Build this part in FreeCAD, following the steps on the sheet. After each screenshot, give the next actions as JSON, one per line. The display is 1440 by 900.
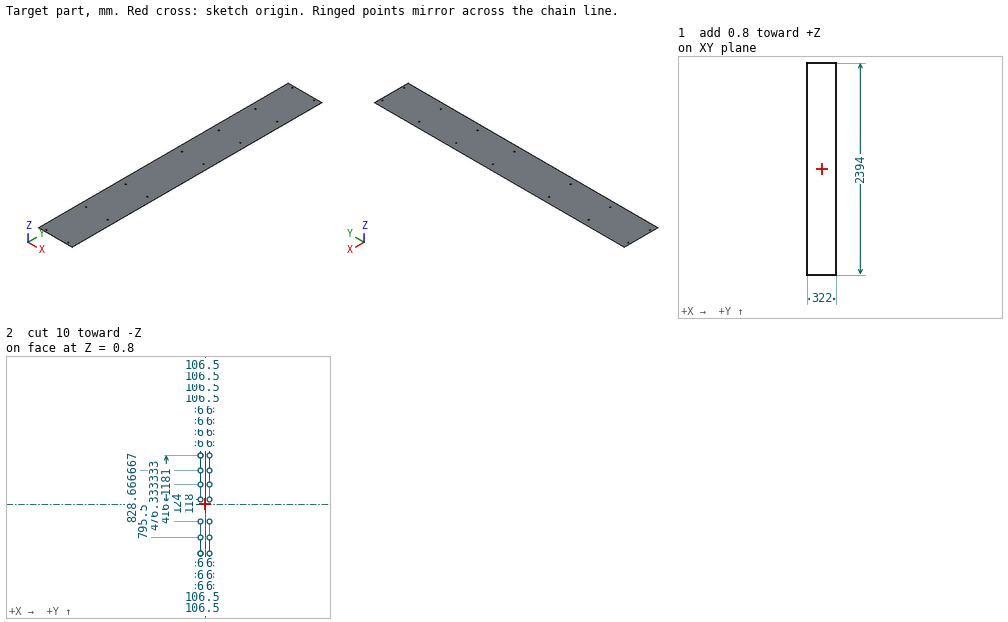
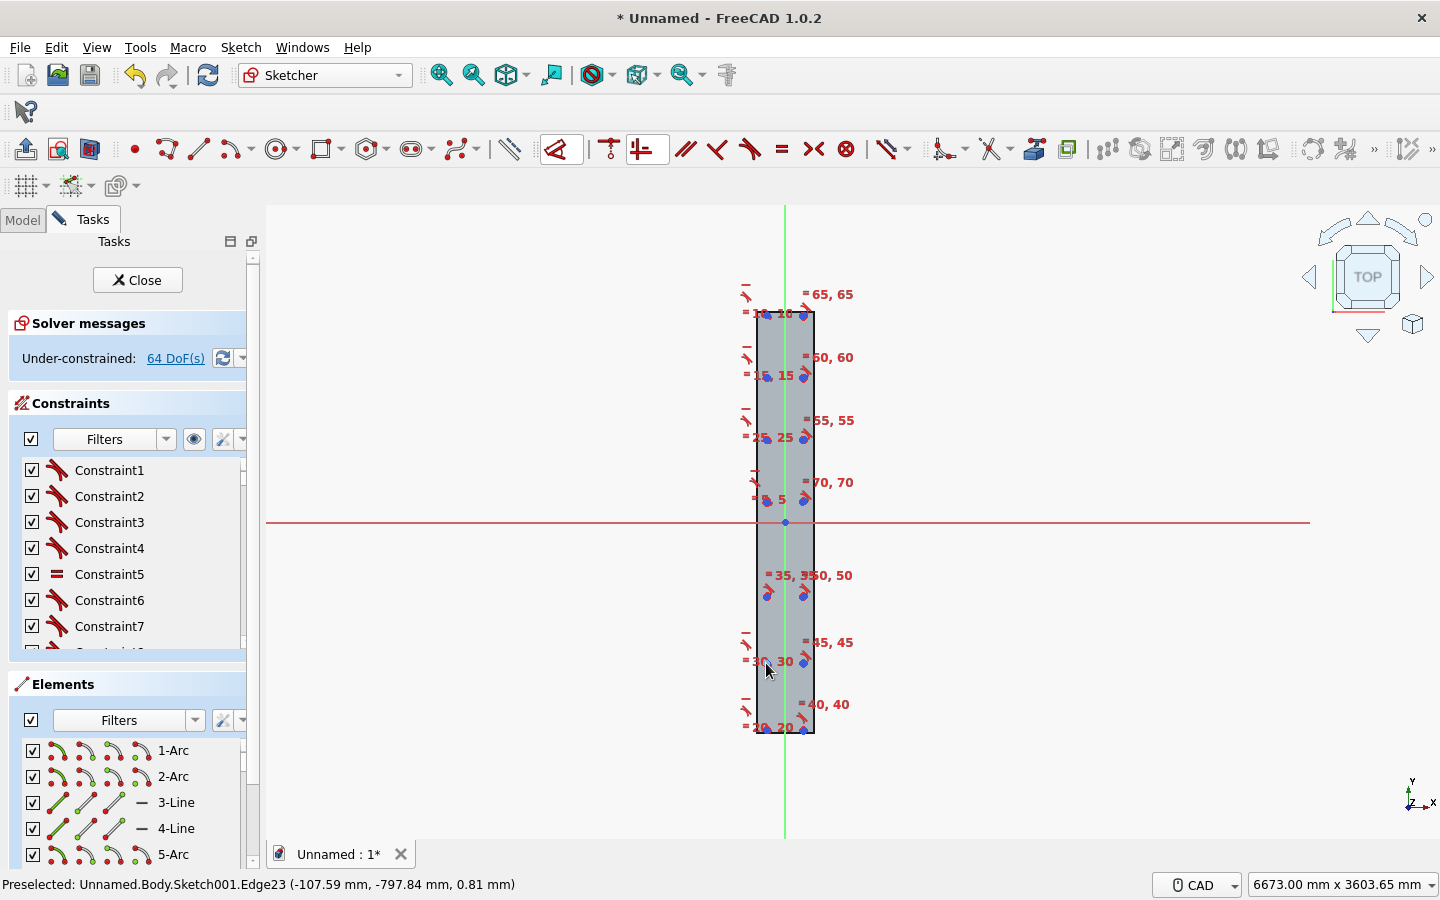
{"action": "scroll", "coordinate": [767, 596], "scroll_direction": "up", "scroll_amount": 14}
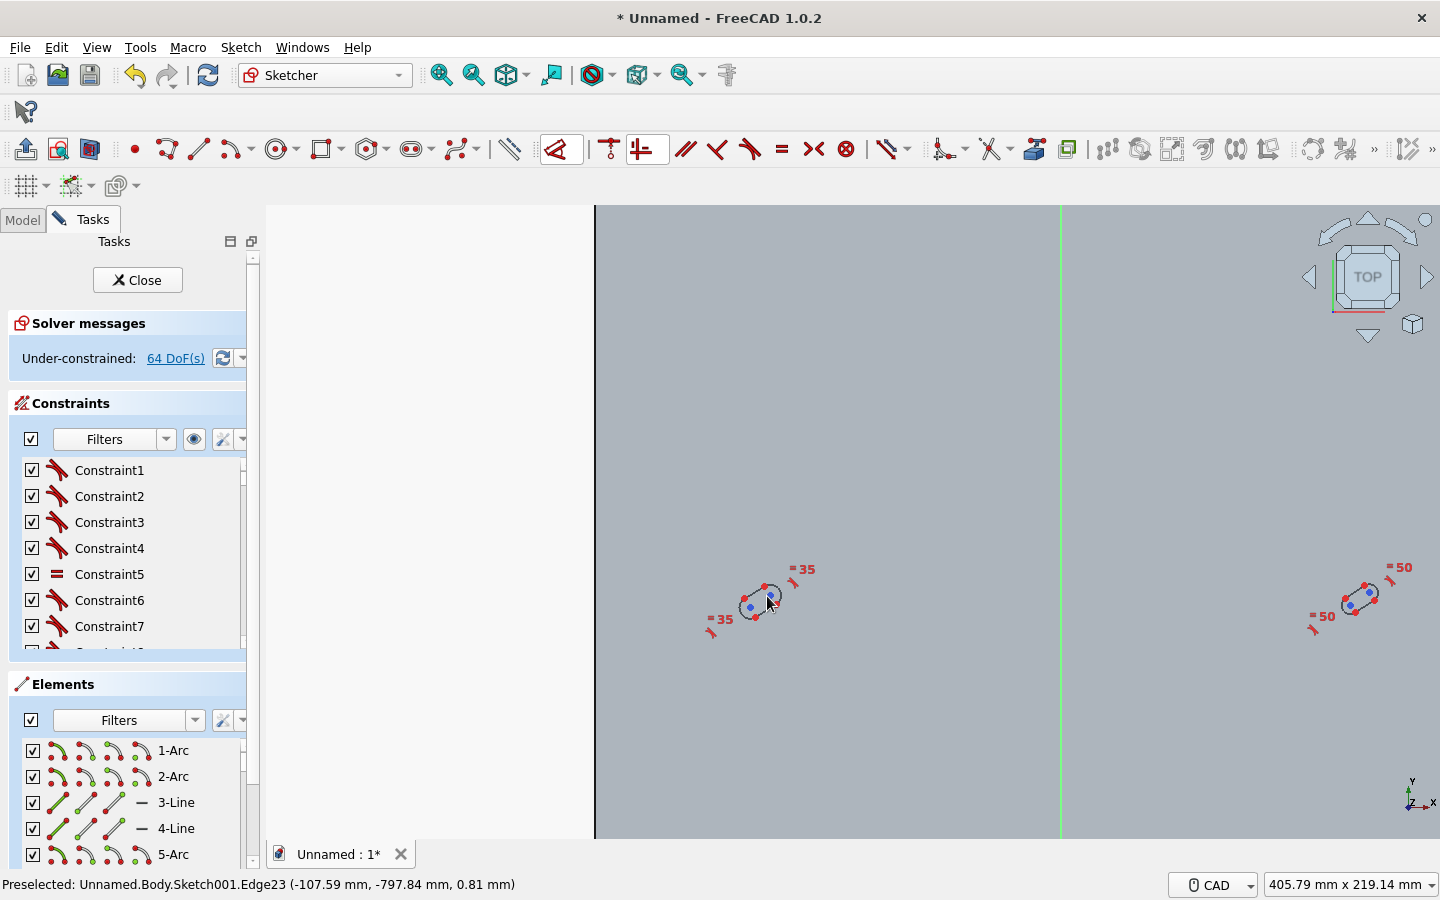
{"action": "left_click", "coordinate": [753, 594]}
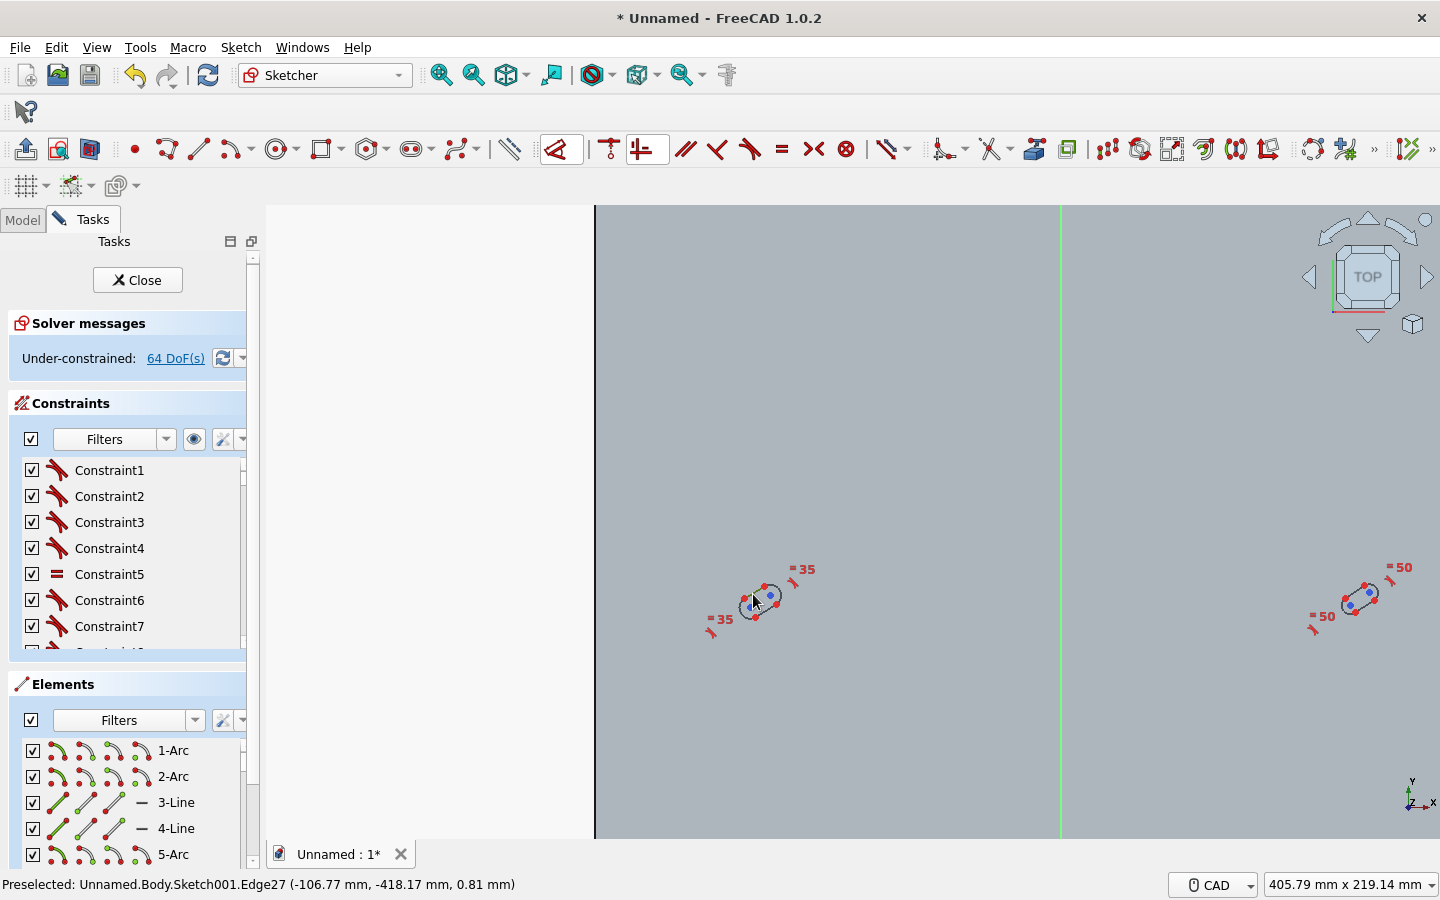
{"action": "key", "text": "h"}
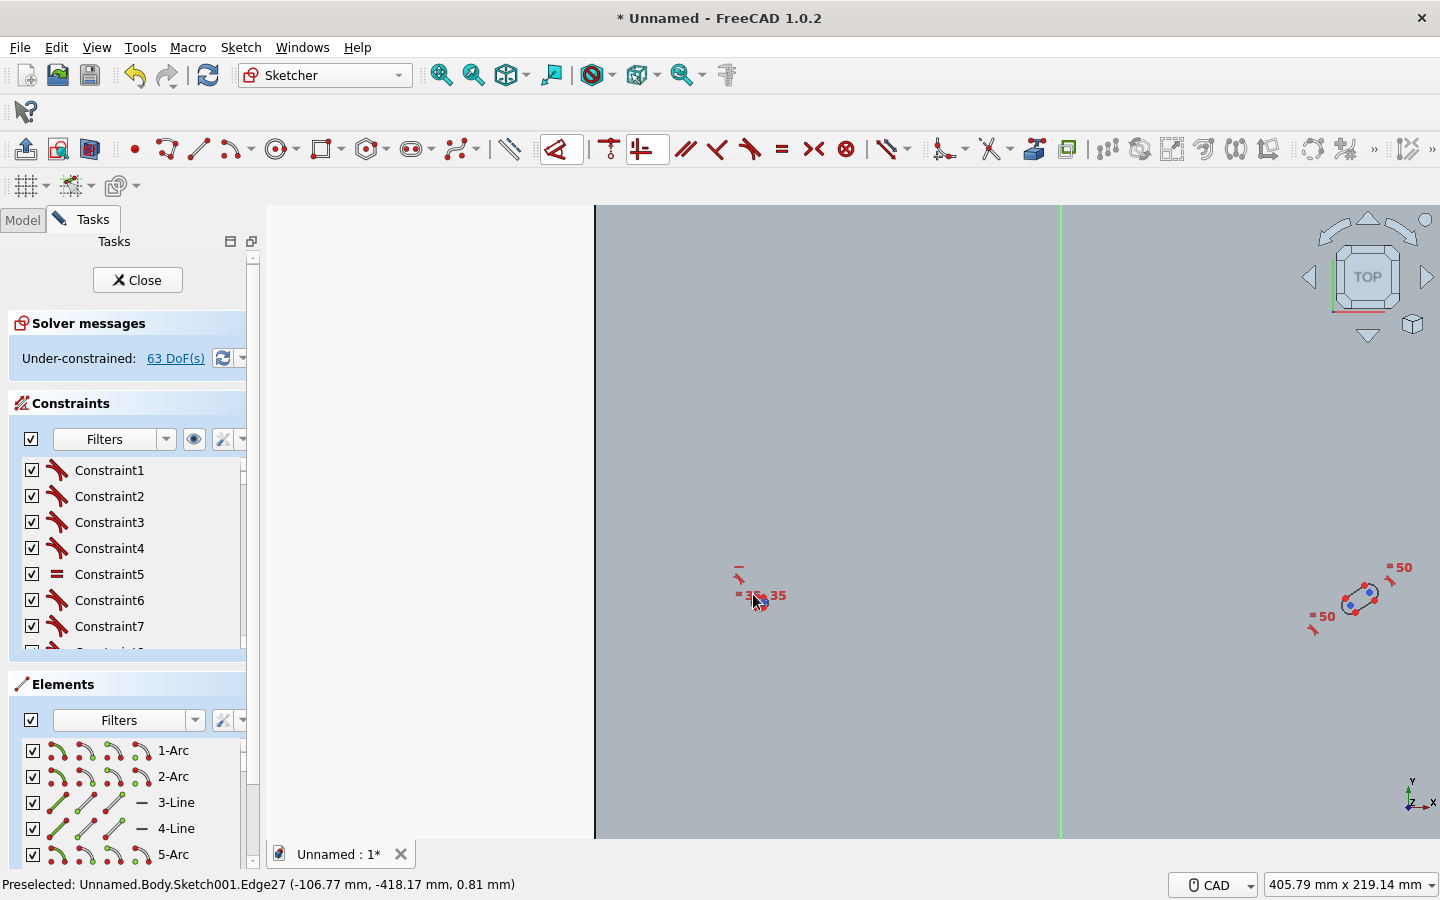
{"action": "scroll", "coordinate": [767, 596], "scroll_direction": "down", "scroll_amount": 14}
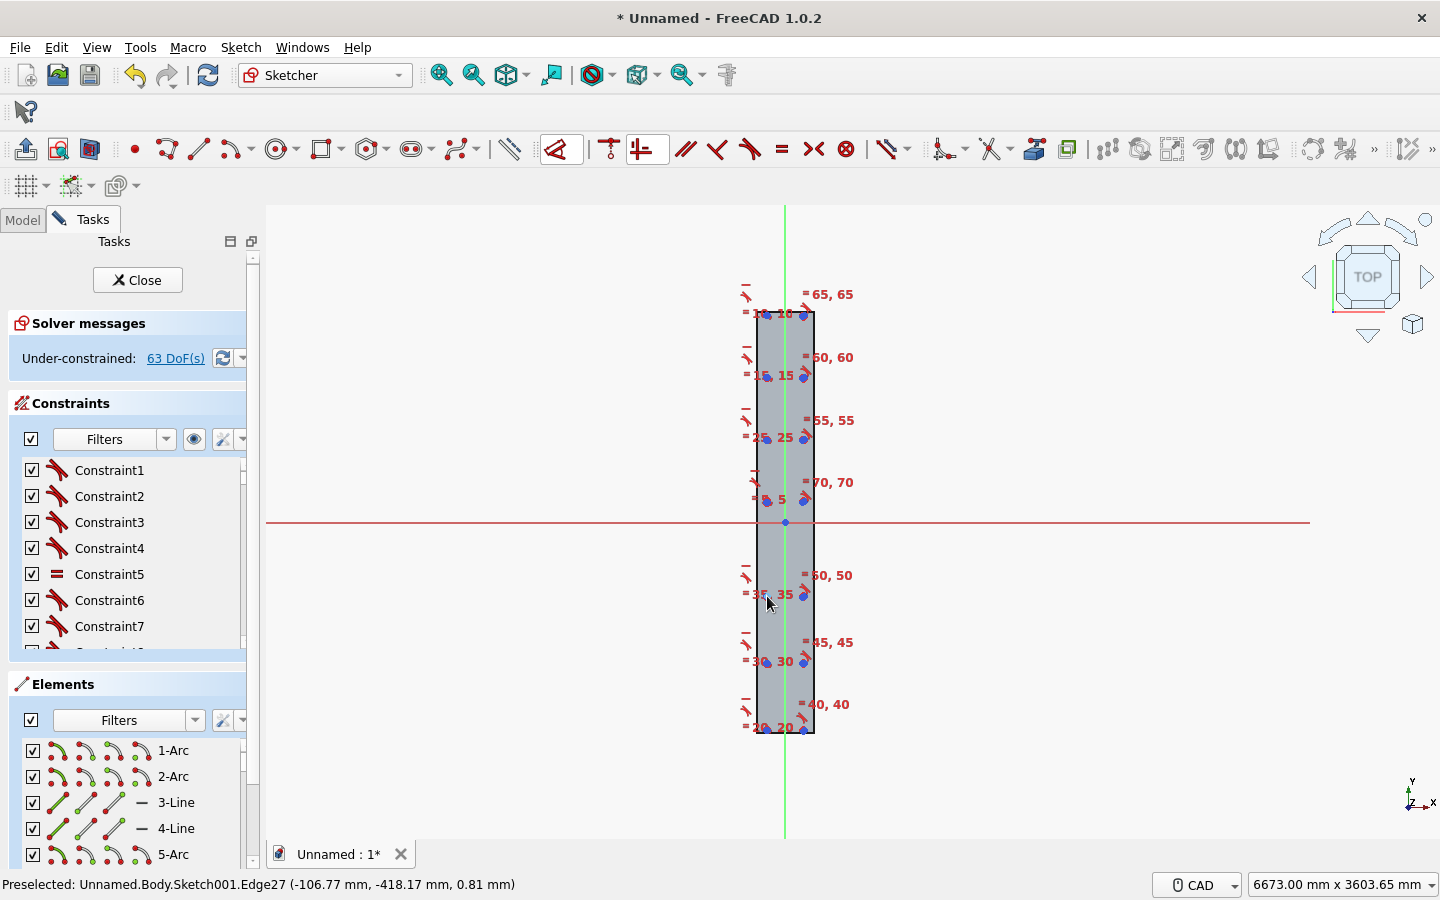
{"action": "scroll", "coordinate": [803, 730], "scroll_direction": "up", "scroll_amount": 14}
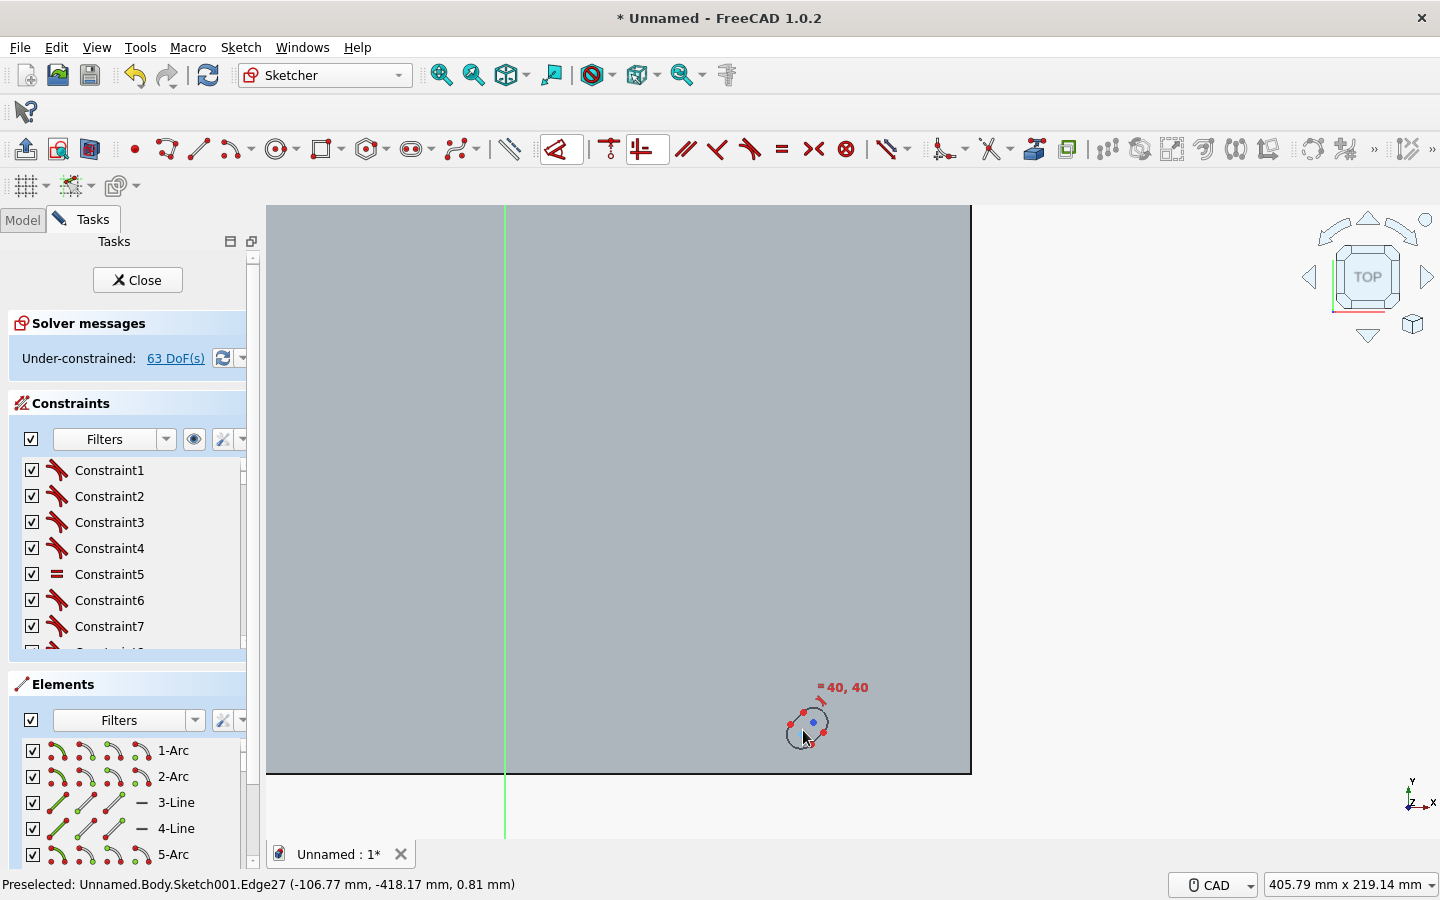
{"action": "left_click", "coordinate": [797, 718]}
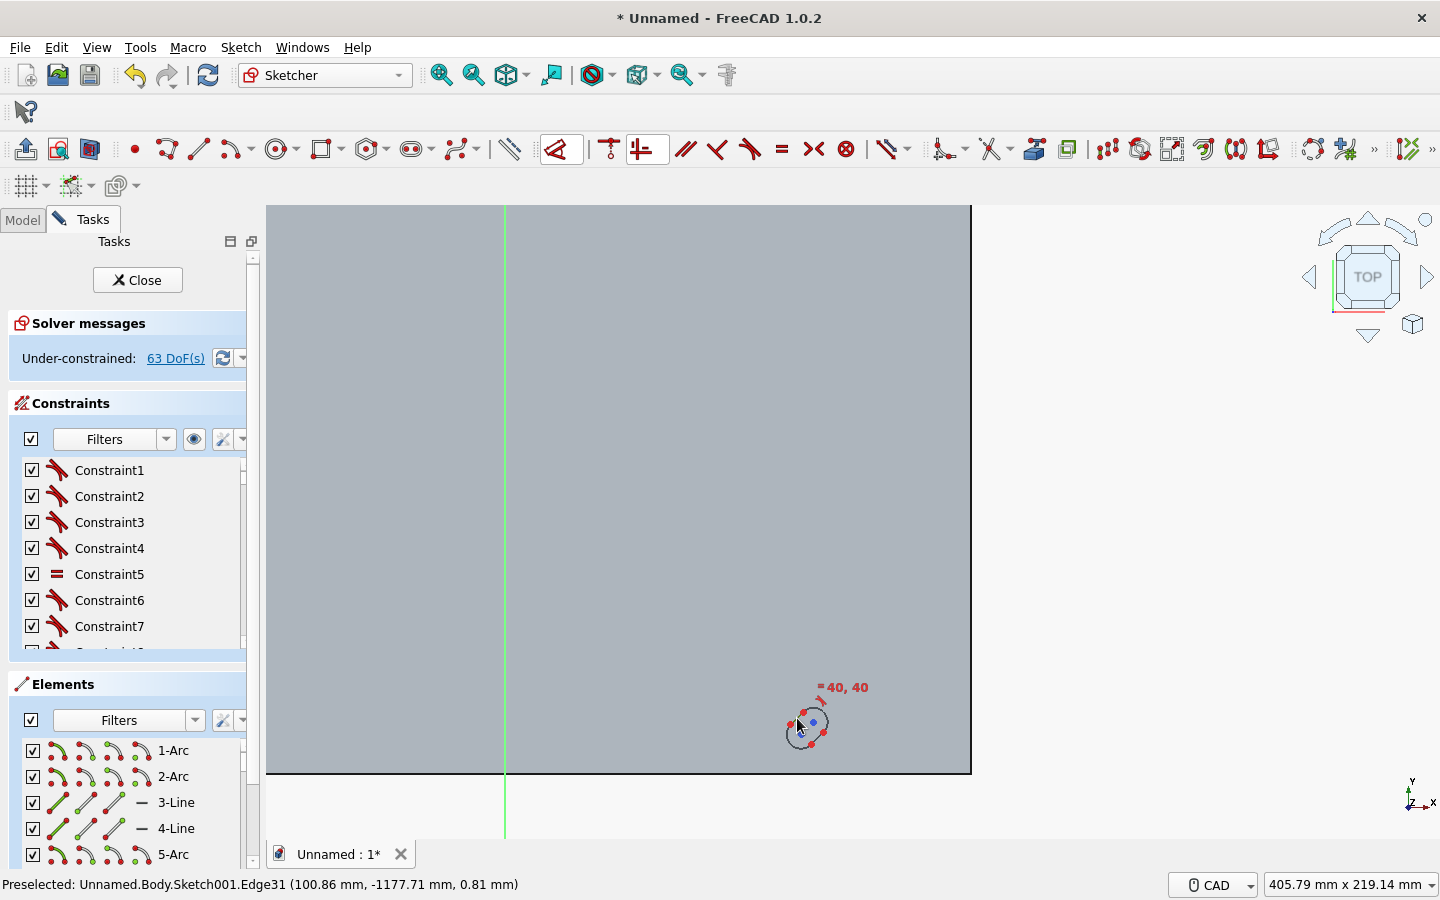
{"action": "key", "text": "h"}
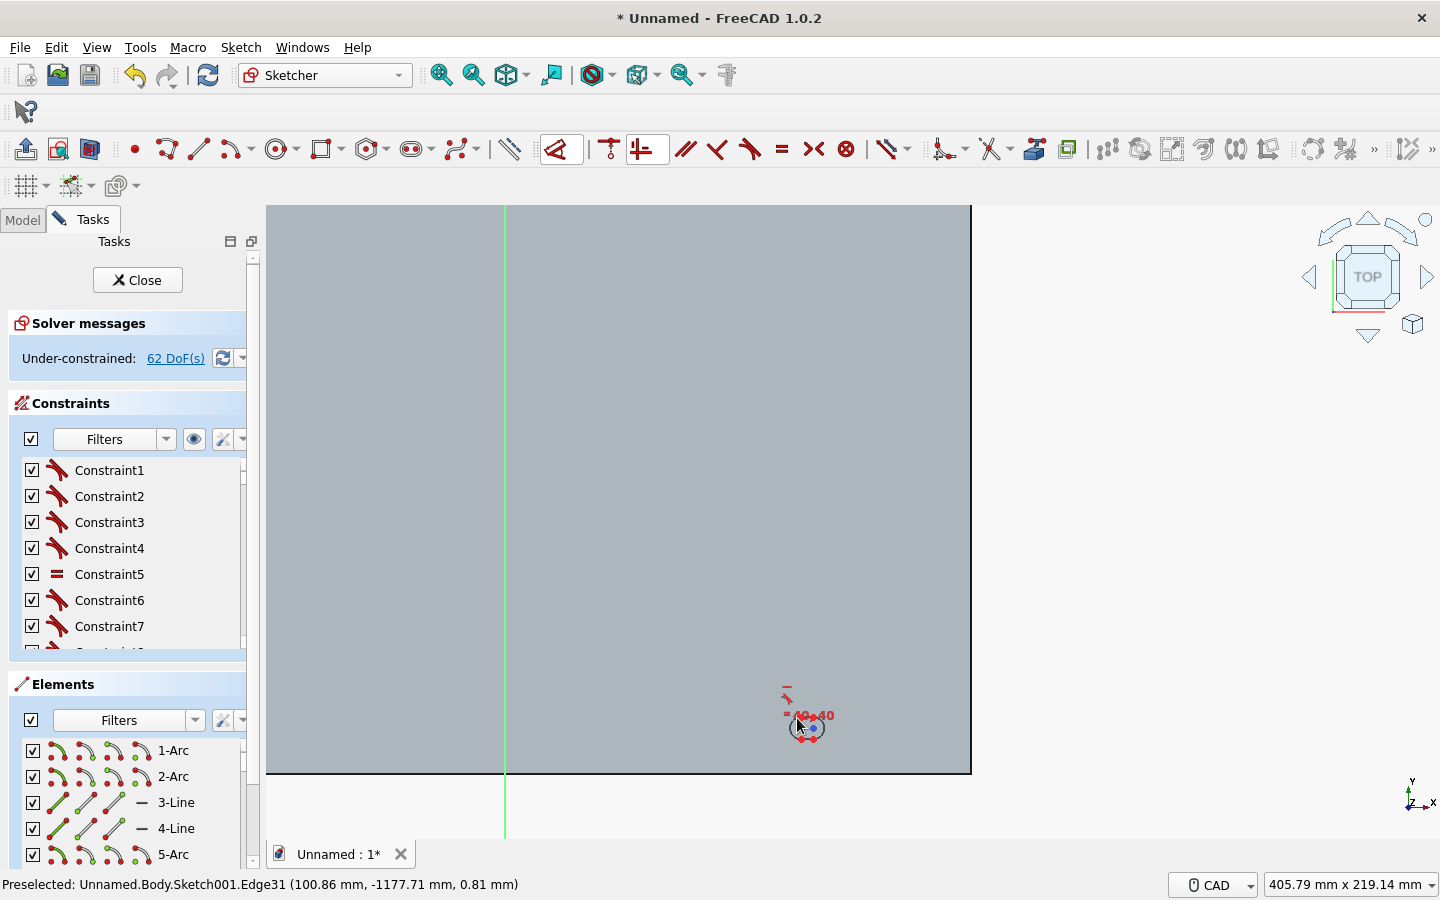
{"action": "scroll", "coordinate": [803, 730], "scroll_direction": "down", "scroll_amount": 14}